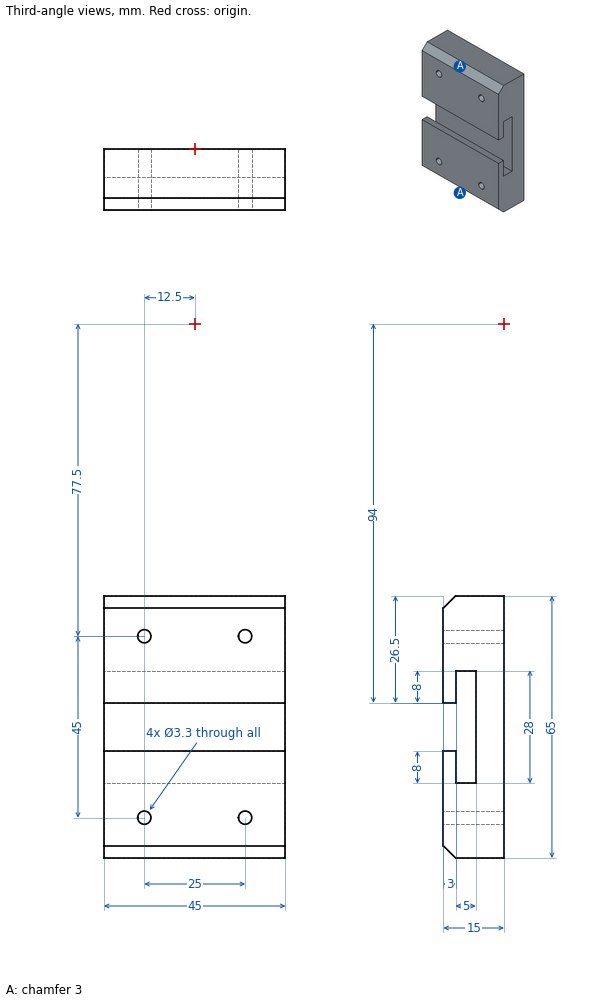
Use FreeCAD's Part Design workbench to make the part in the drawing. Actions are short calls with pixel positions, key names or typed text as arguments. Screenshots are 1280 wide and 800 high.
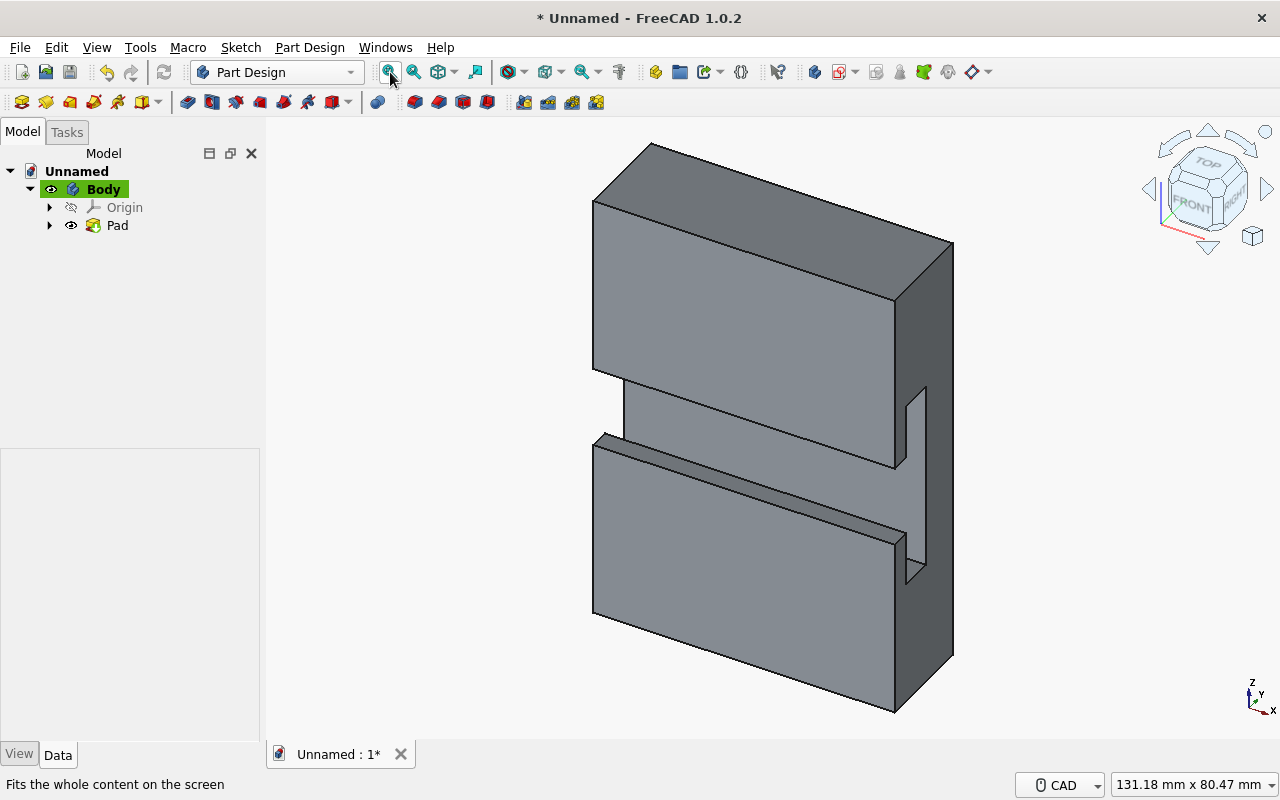
click(744, 250)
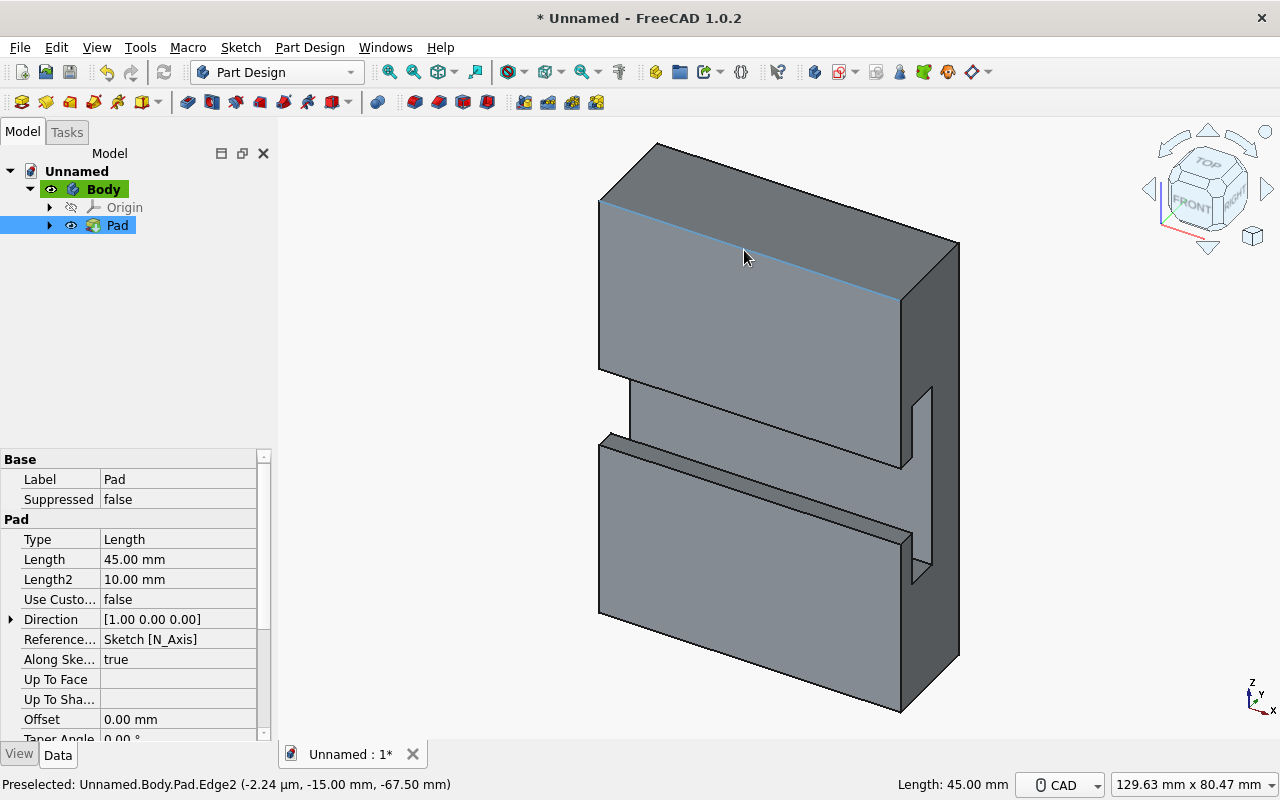
key(0)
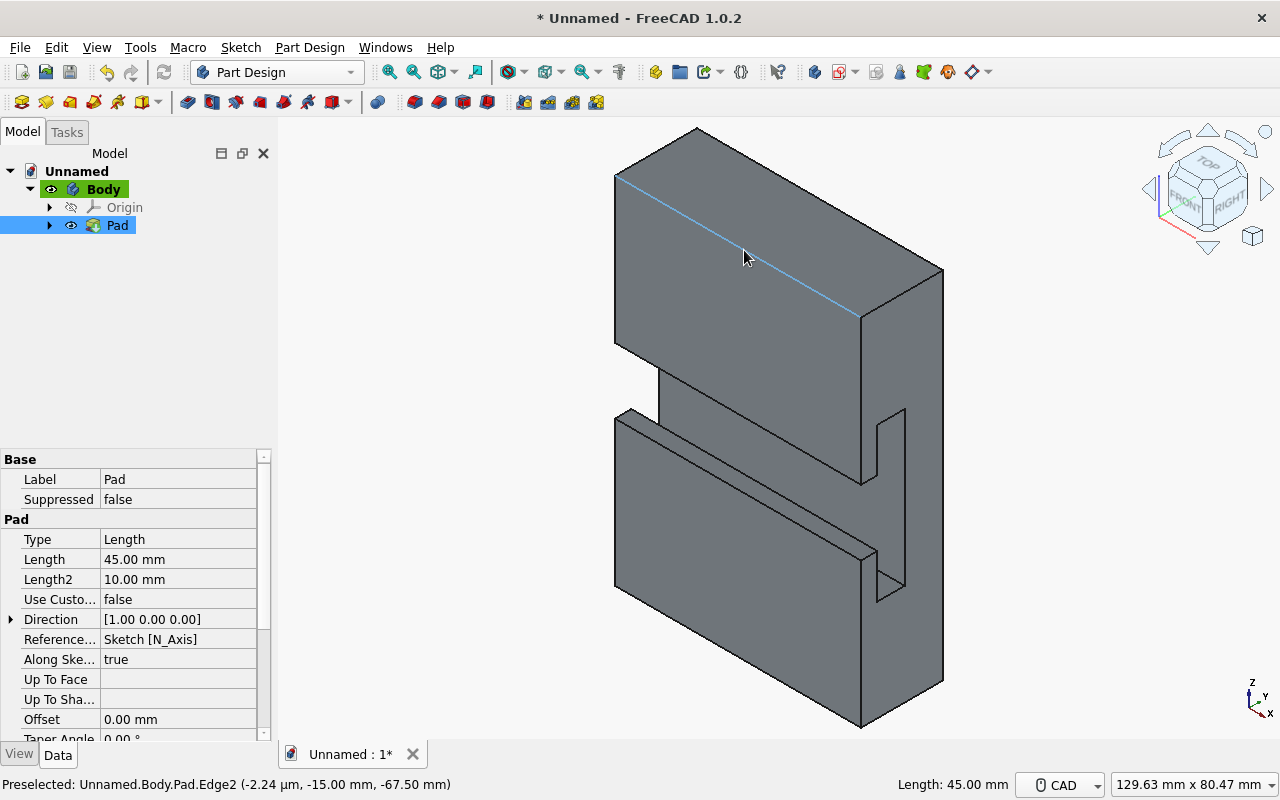
key(2)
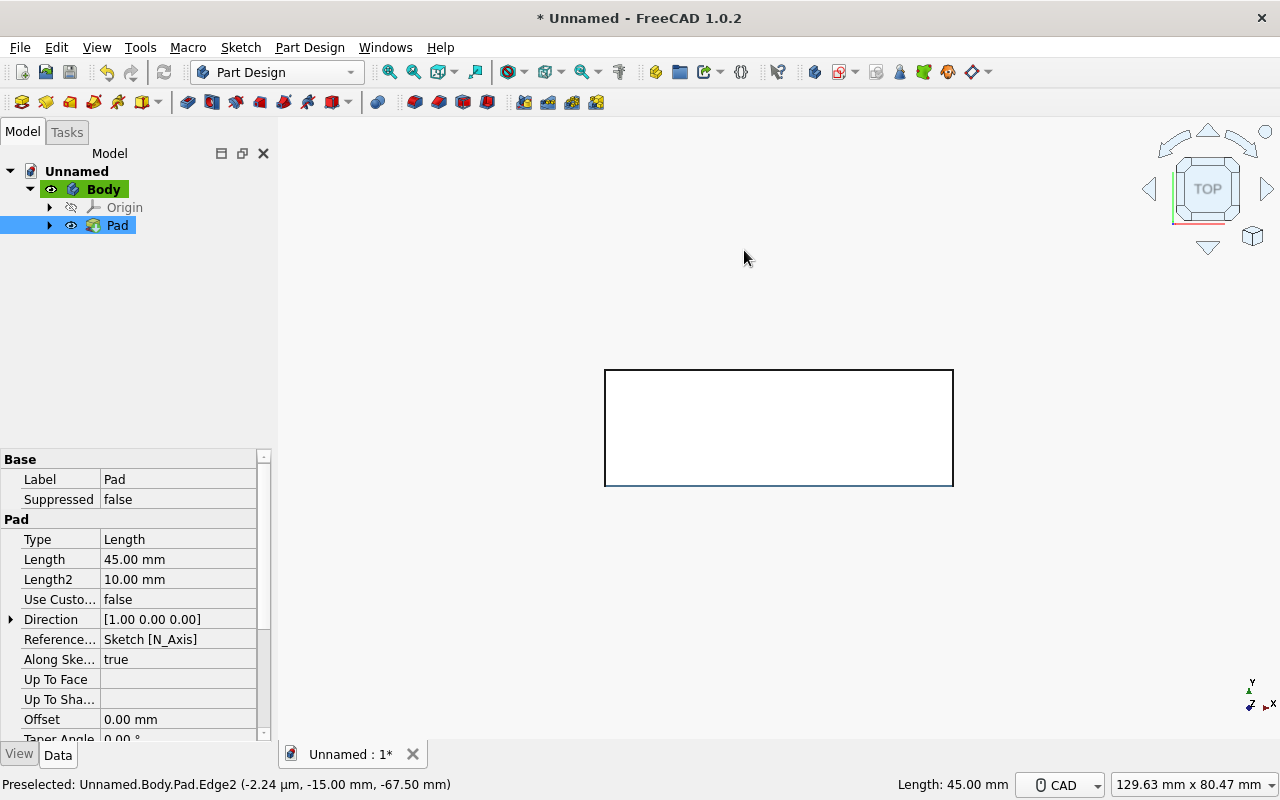
click(390, 72)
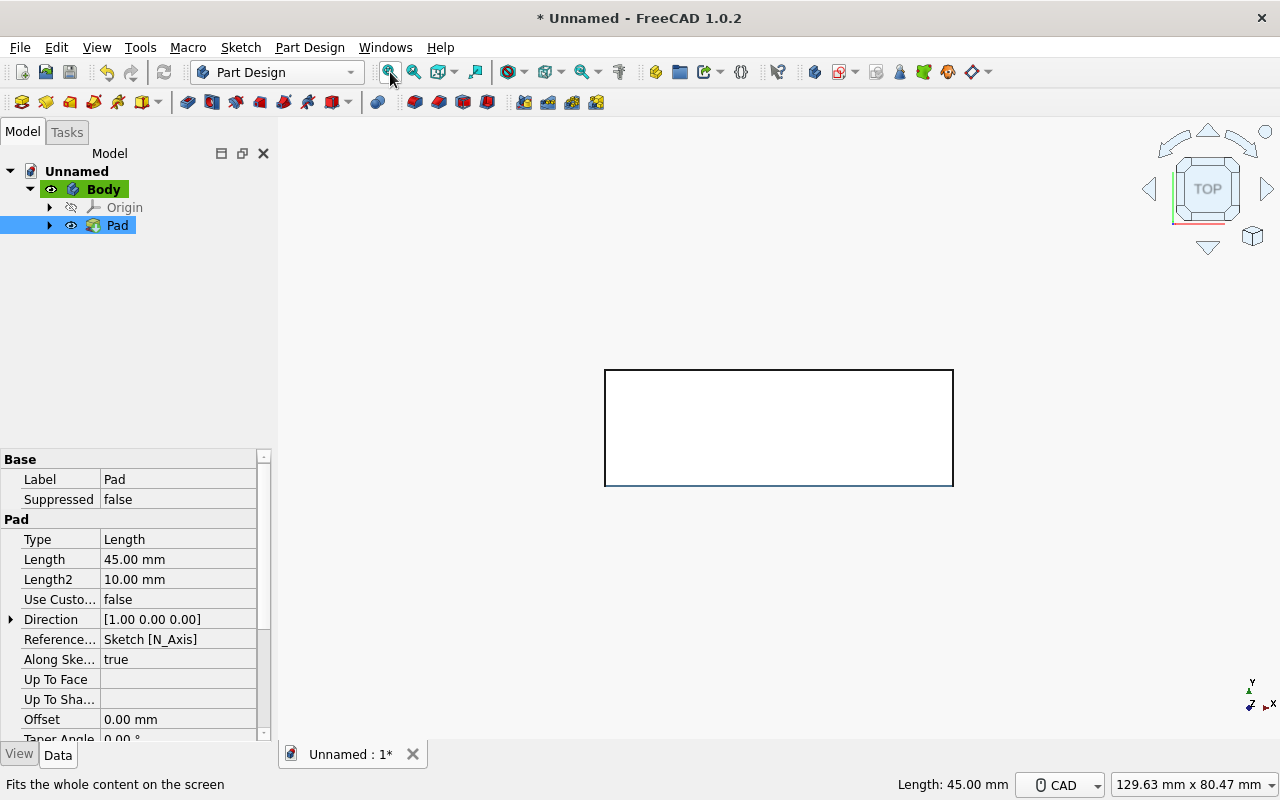
key(1)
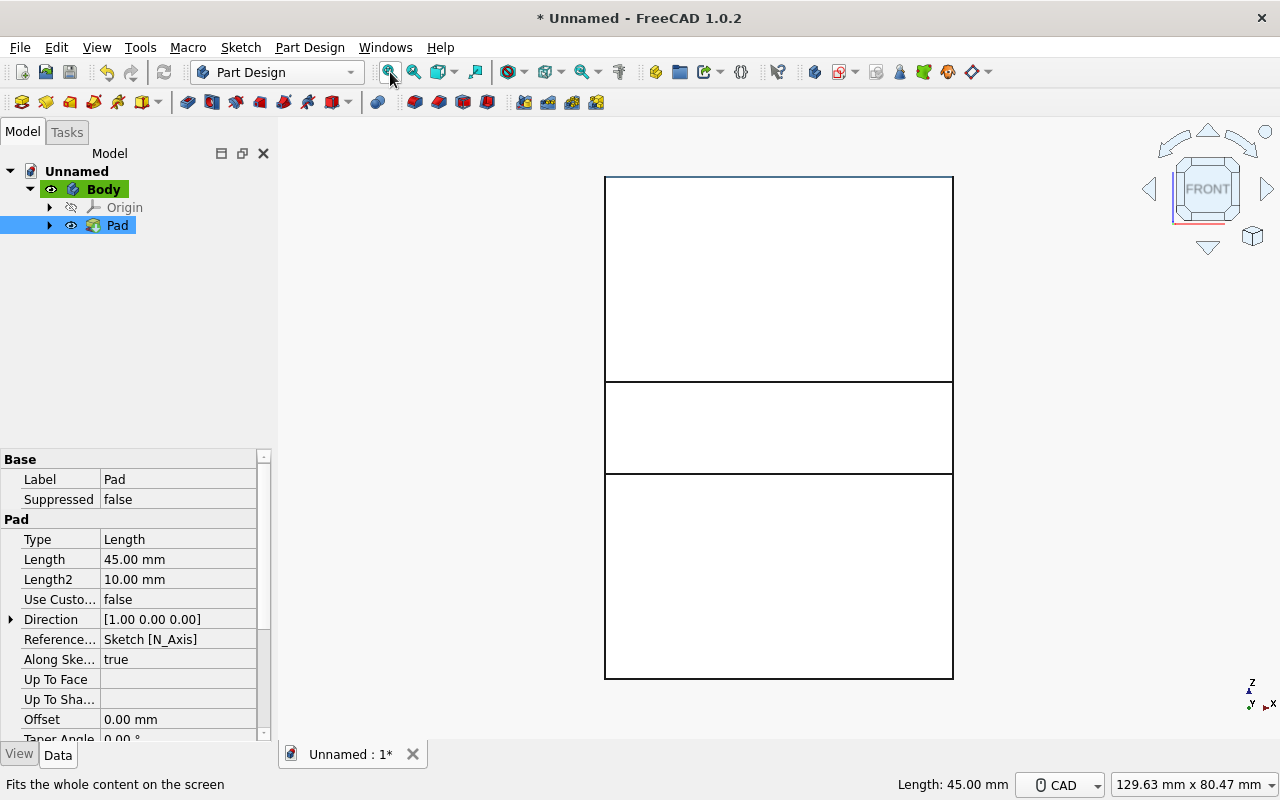
click(779, 678, ctrl)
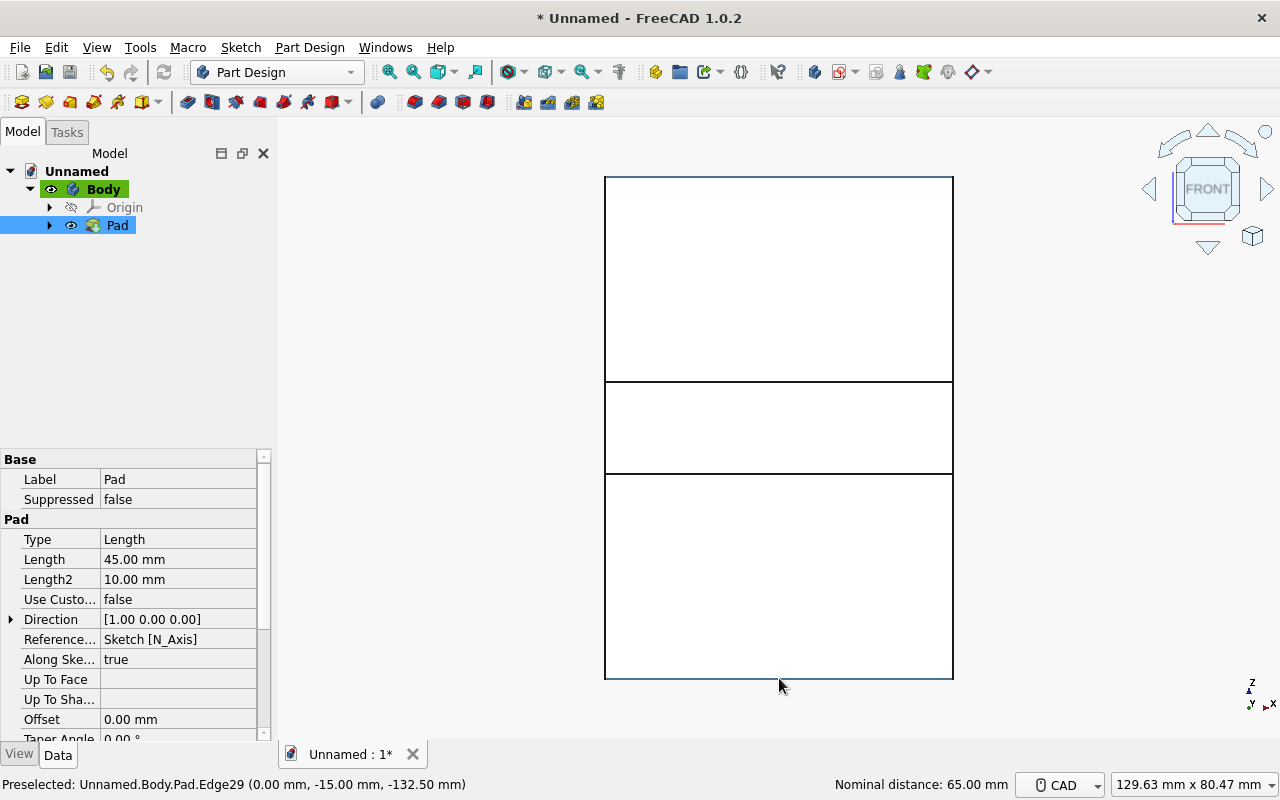
click(440, 102)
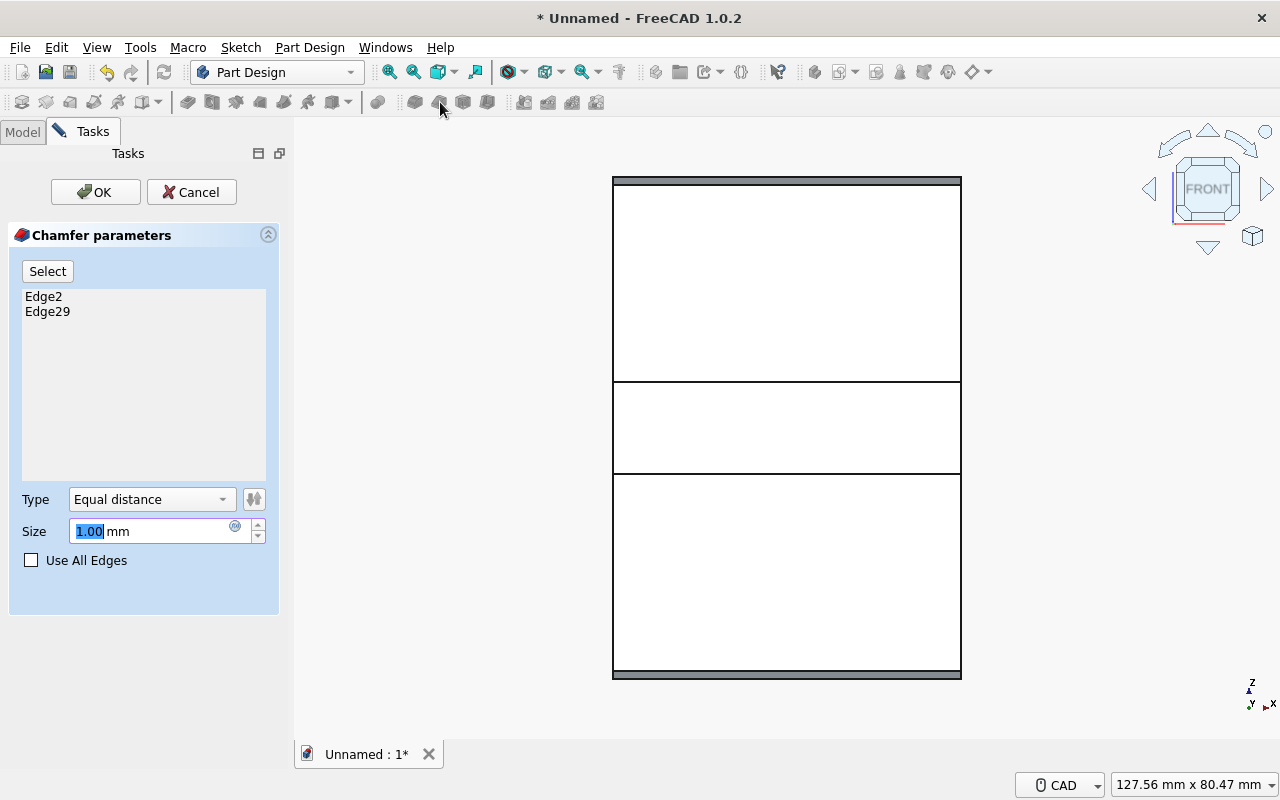
text(3)
key(Tab)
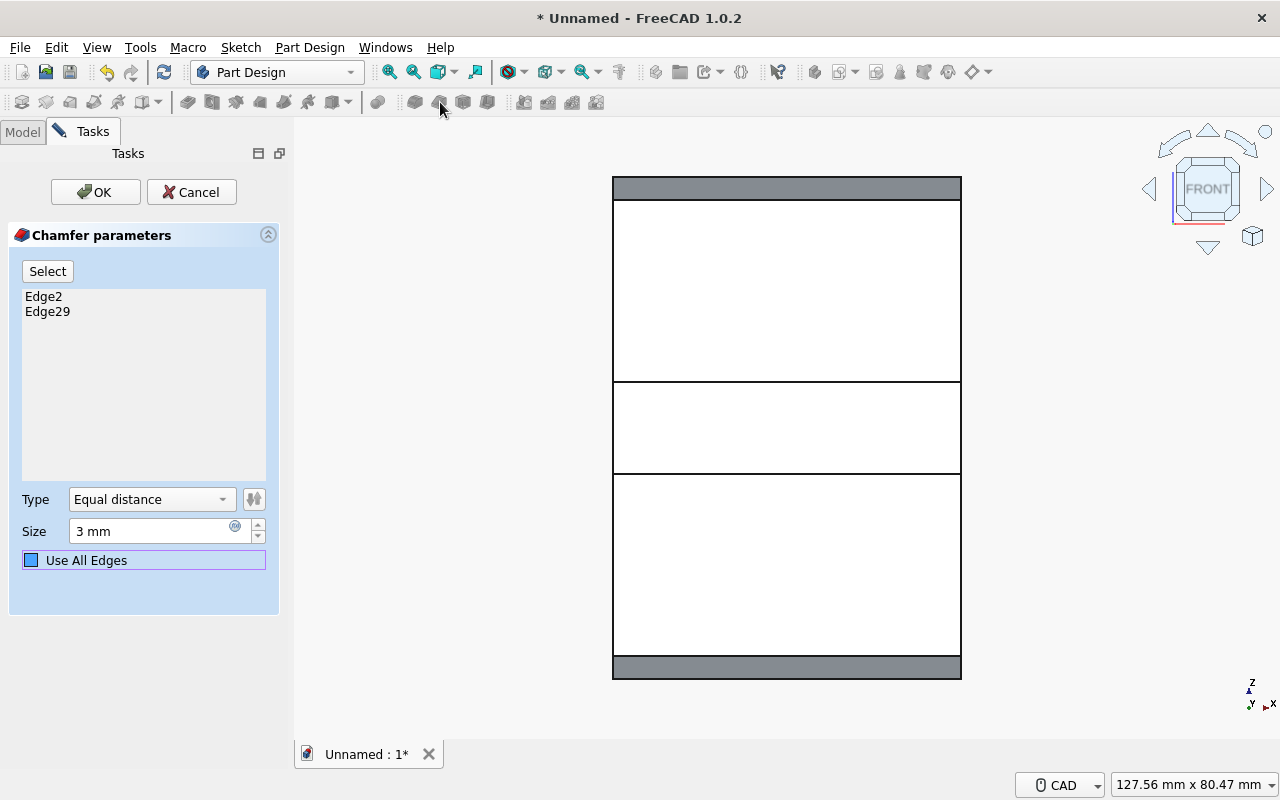
click(96, 192)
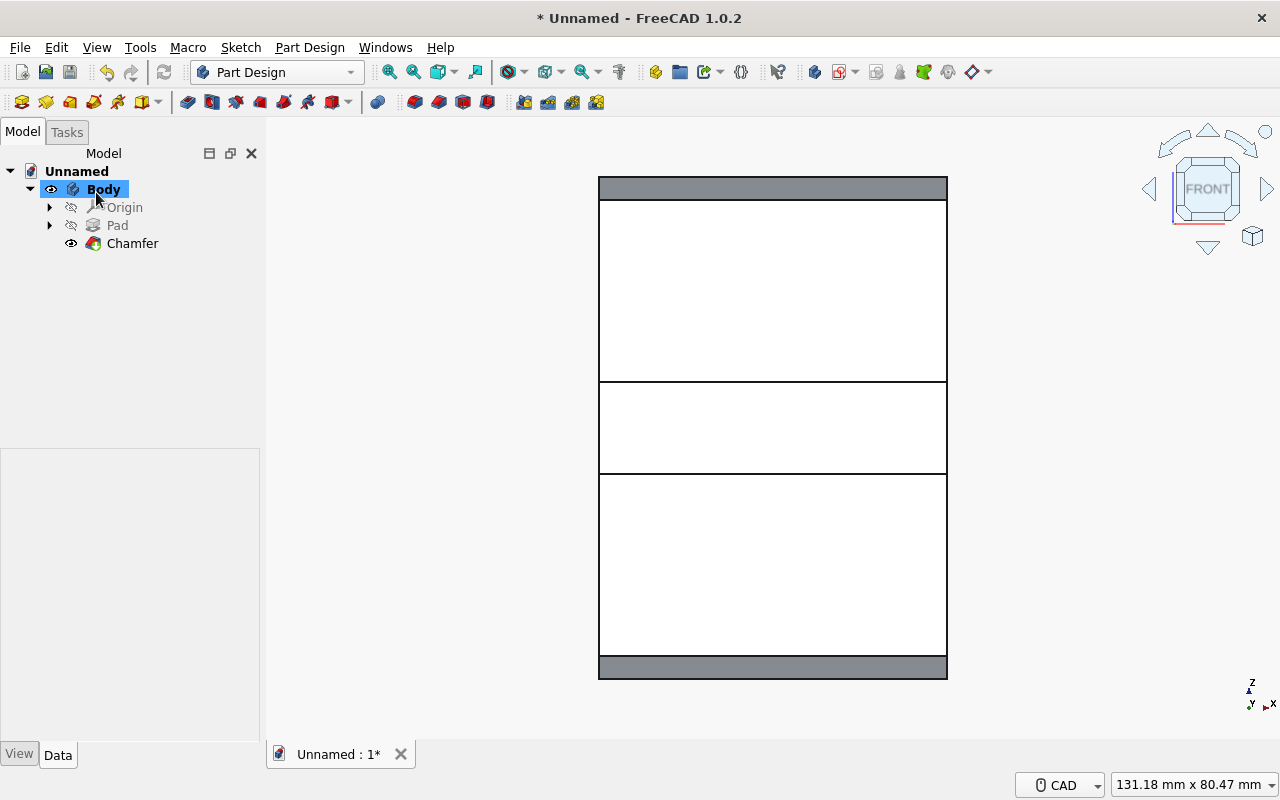
key(4)